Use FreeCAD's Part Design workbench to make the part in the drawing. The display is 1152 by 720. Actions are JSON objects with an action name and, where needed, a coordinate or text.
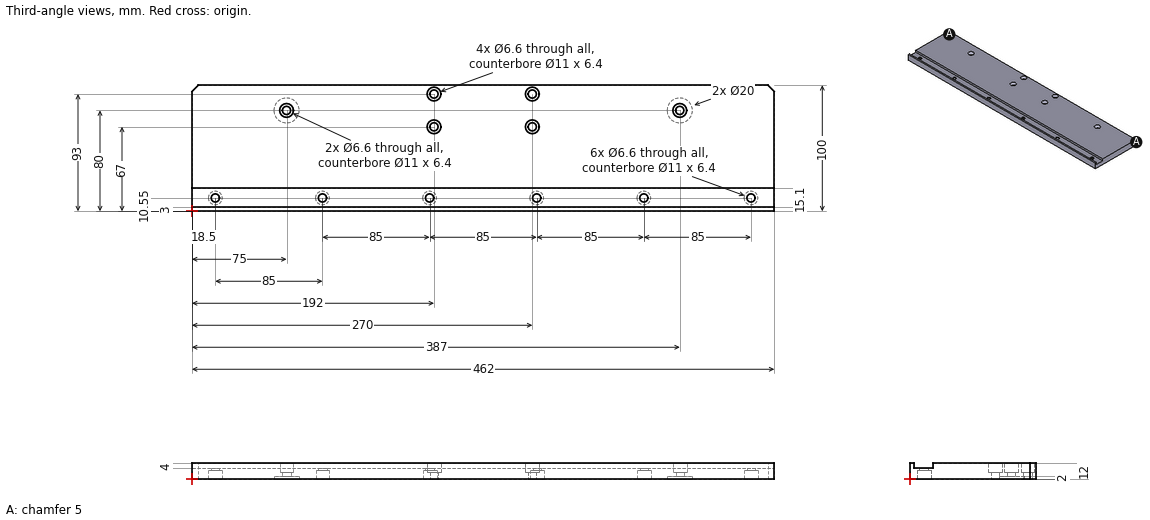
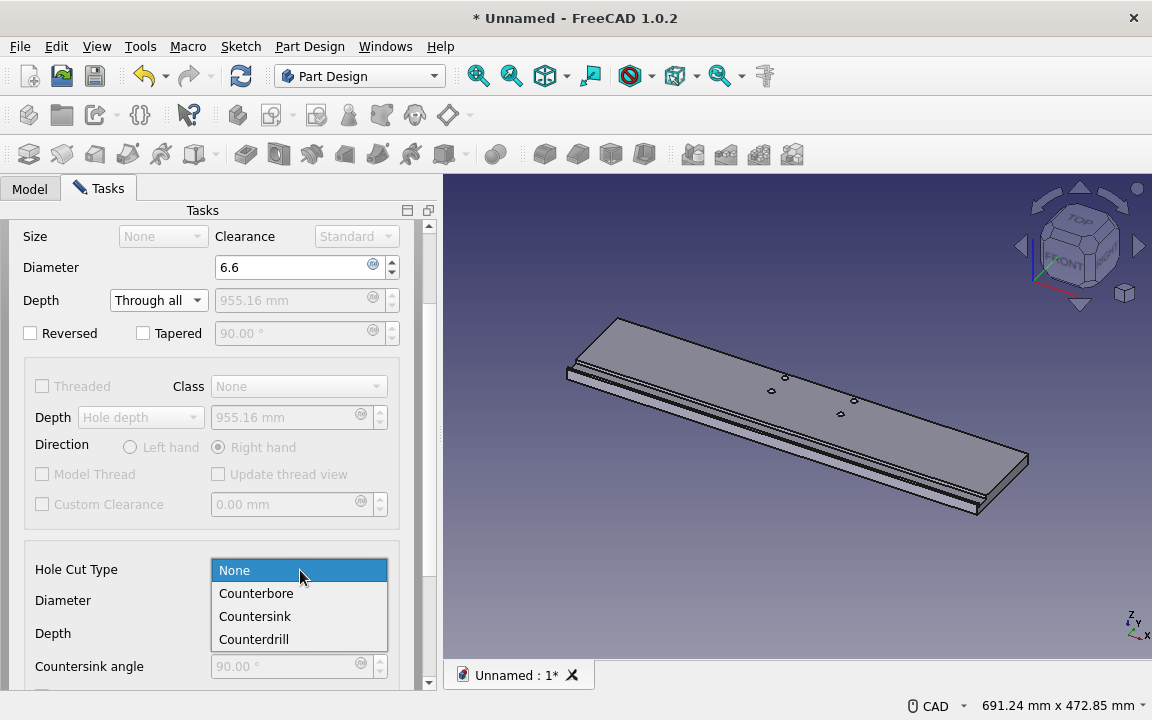
{"action": "left_click", "coordinate": [298, 594]}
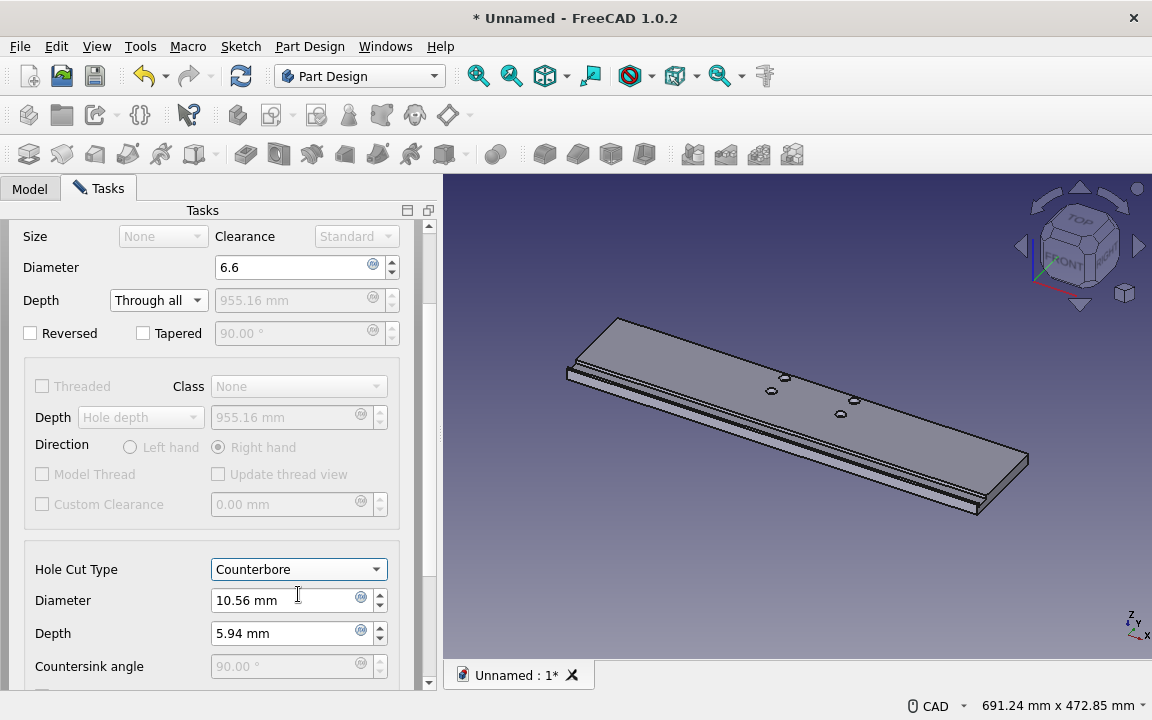
{"action": "triple_click", "coordinate": [292, 600]}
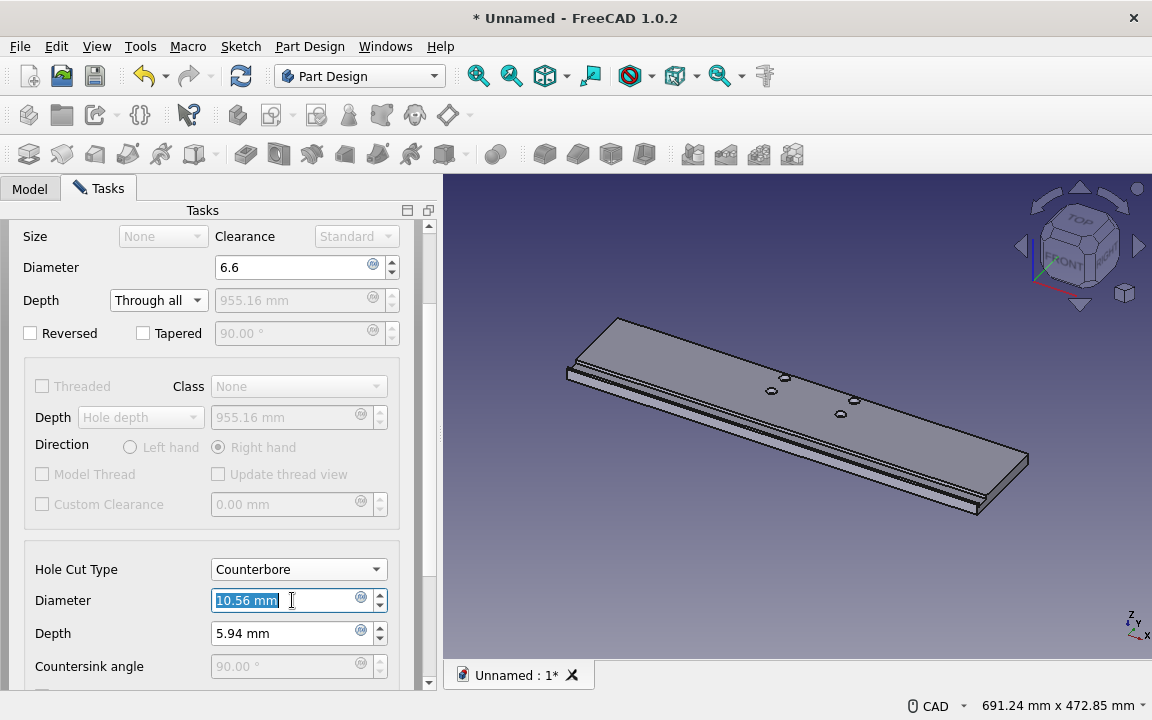
{"action": "type", "text": "11"}
{"action": "key", "text": "Tab"}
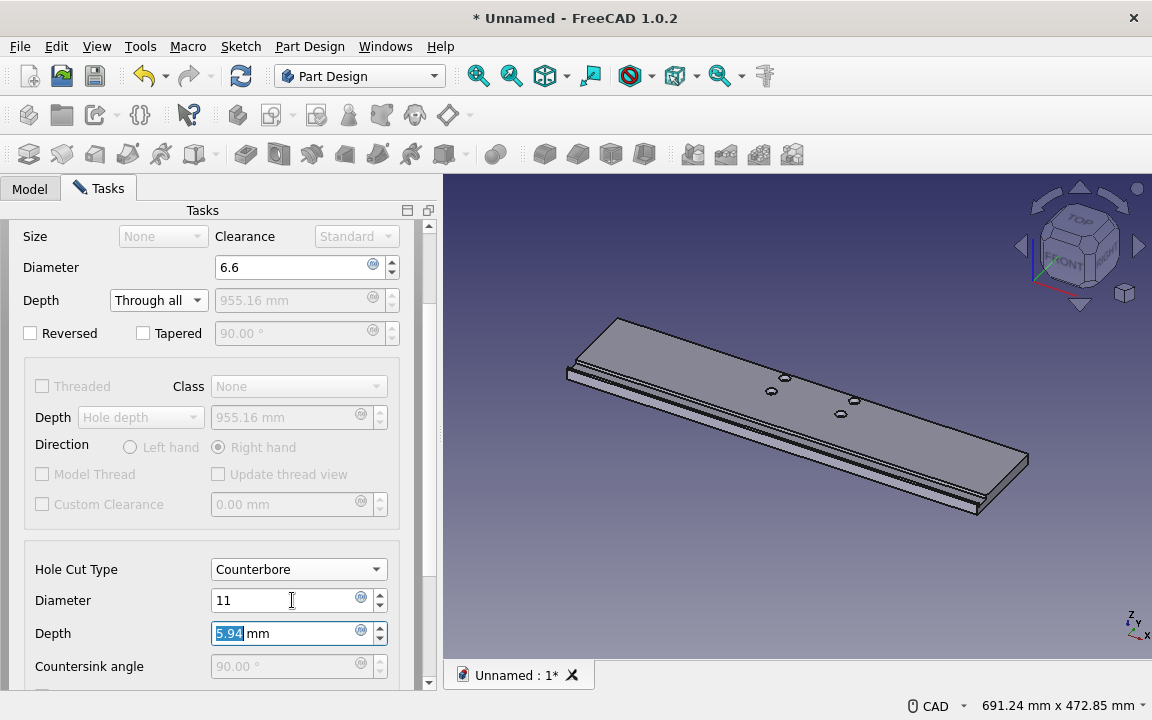
{"action": "type", "text": "6.4"}
{"action": "key", "text": "Tab"}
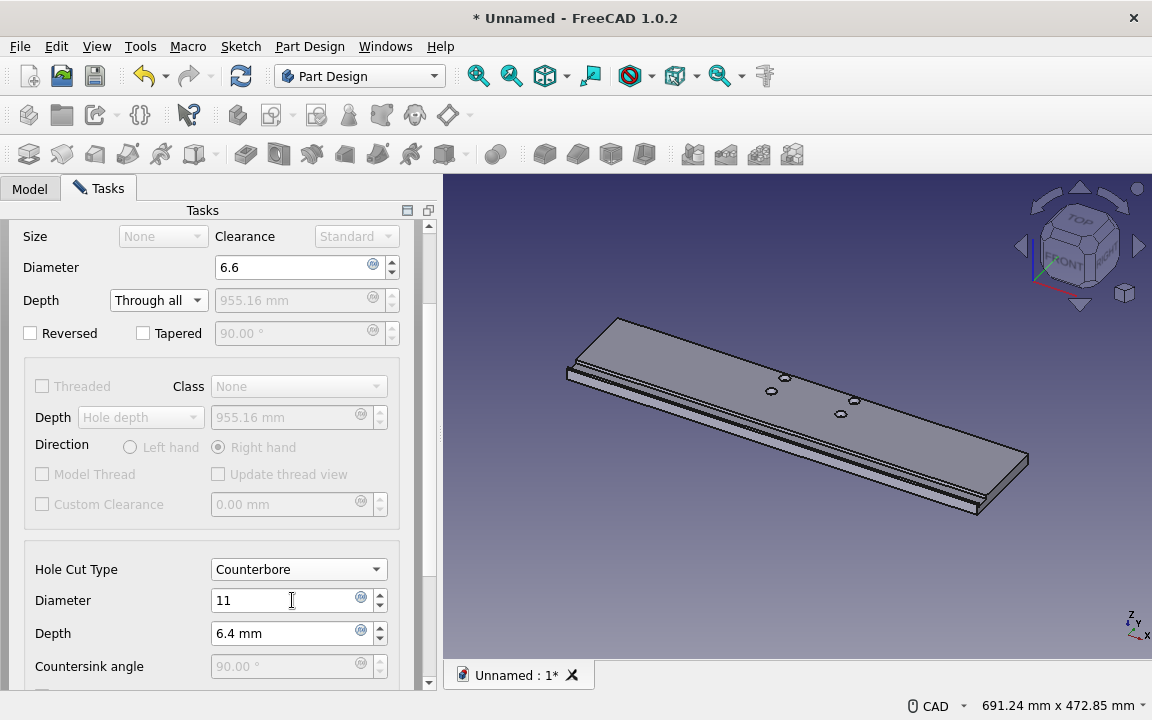
{"action": "scroll", "coordinate": [429, 455], "scroll_direction": "up", "scroll_amount": 3}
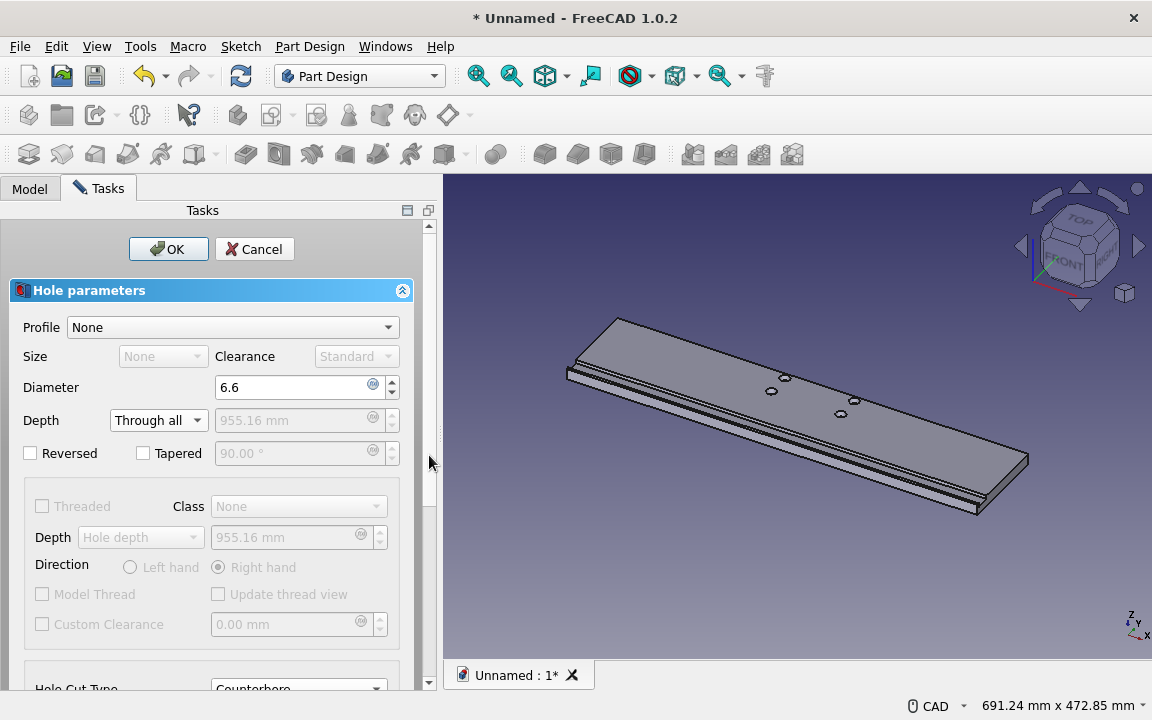
{"action": "left_click", "coordinate": [169, 249]}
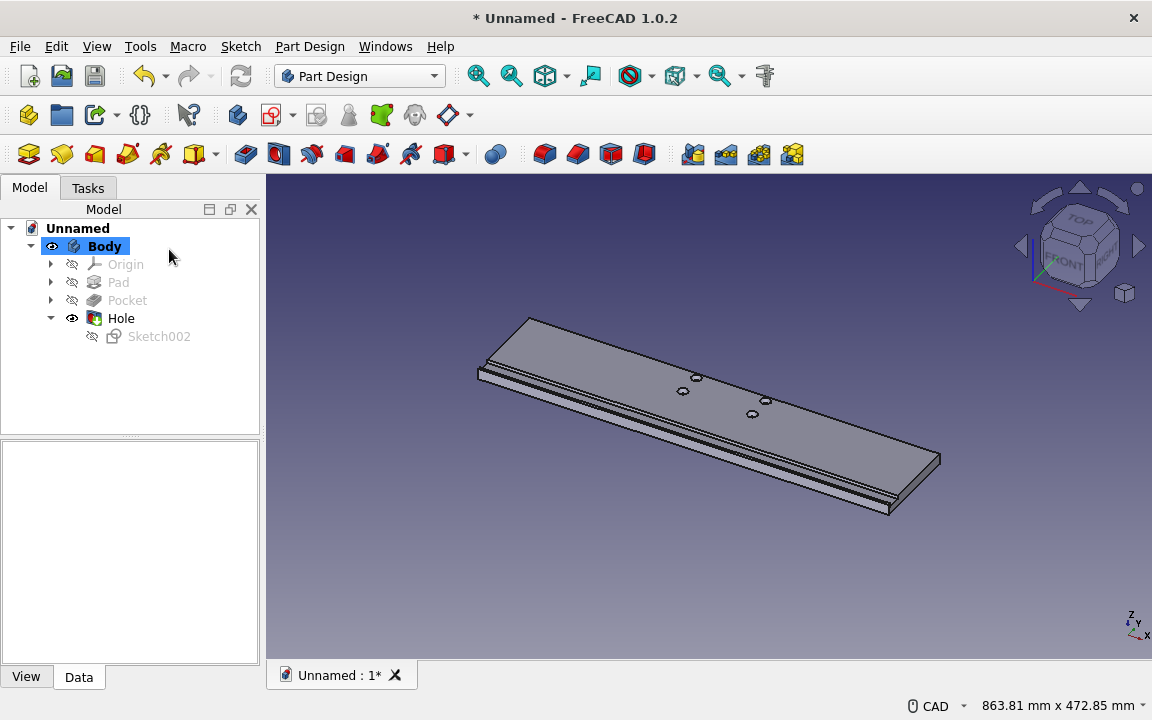
{"action": "left_click", "coordinate": [270, 116]}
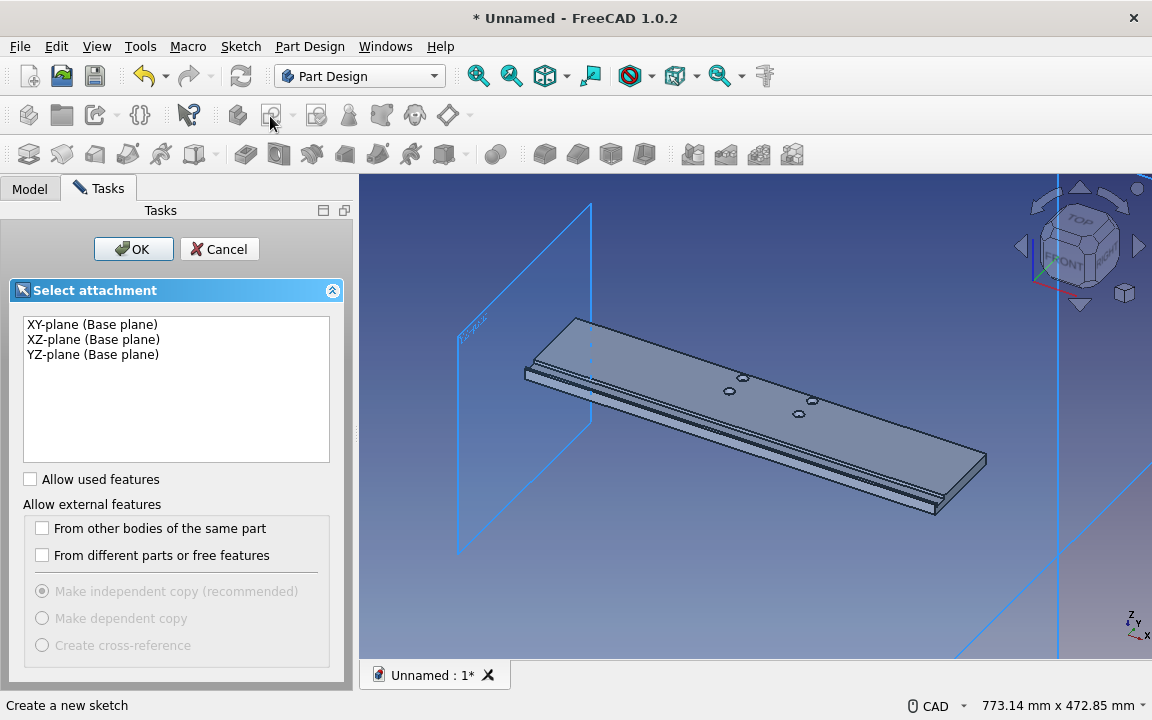
{"action": "left_click", "coordinate": [84, 324]}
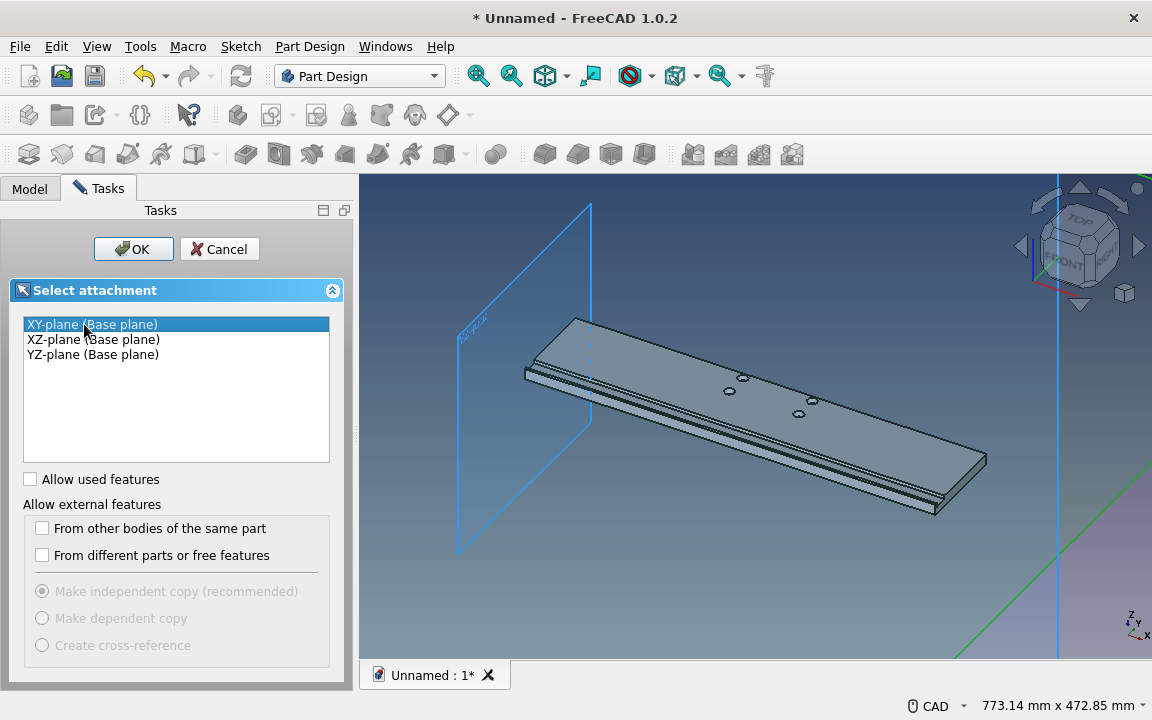
{"action": "left_click", "coordinate": [134, 249]}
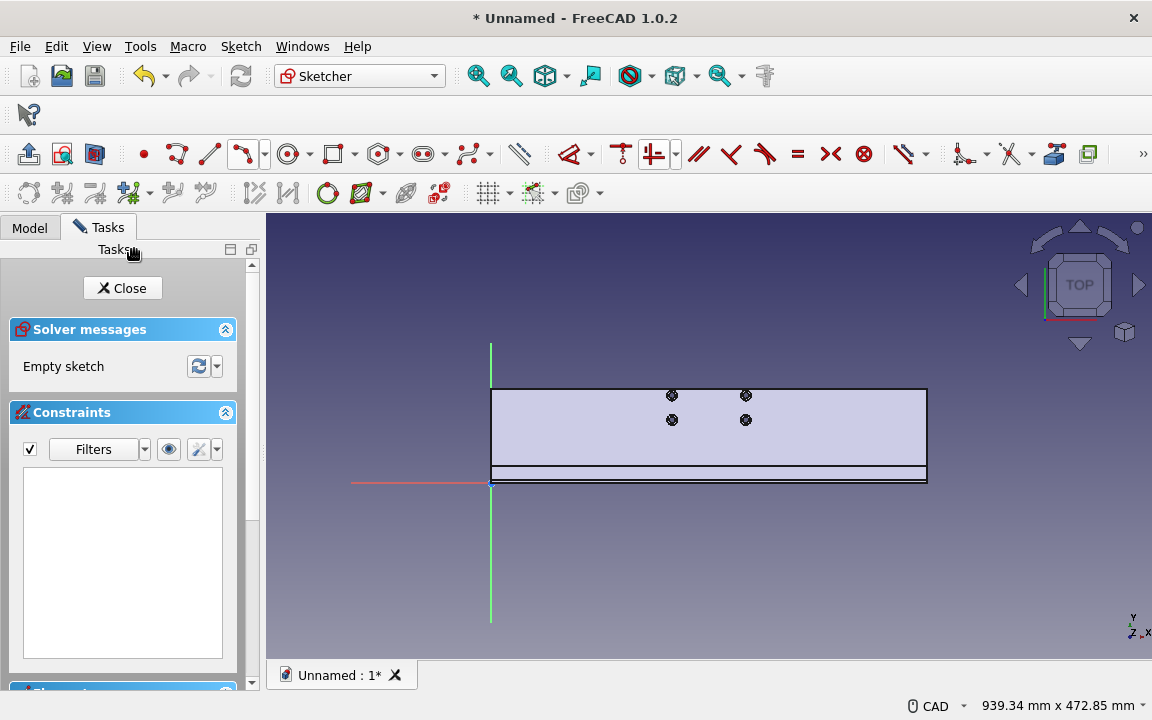
{"action": "left_click", "coordinate": [95, 154]}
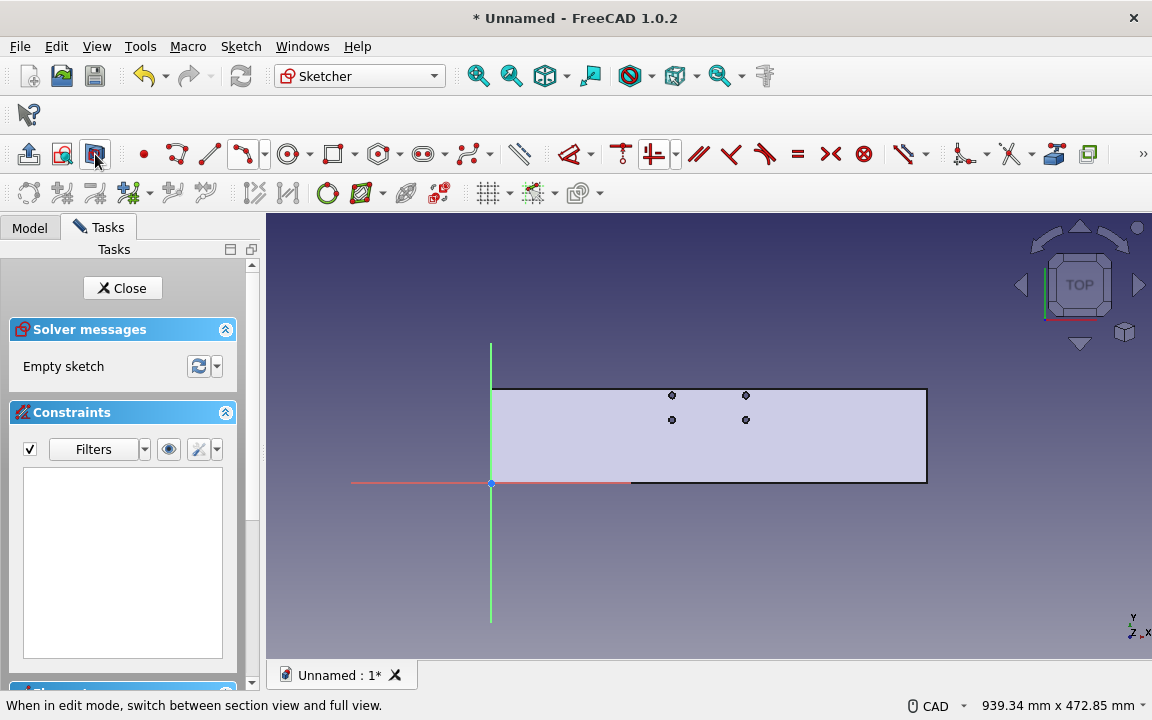
{"action": "left_click", "coordinate": [288, 154]}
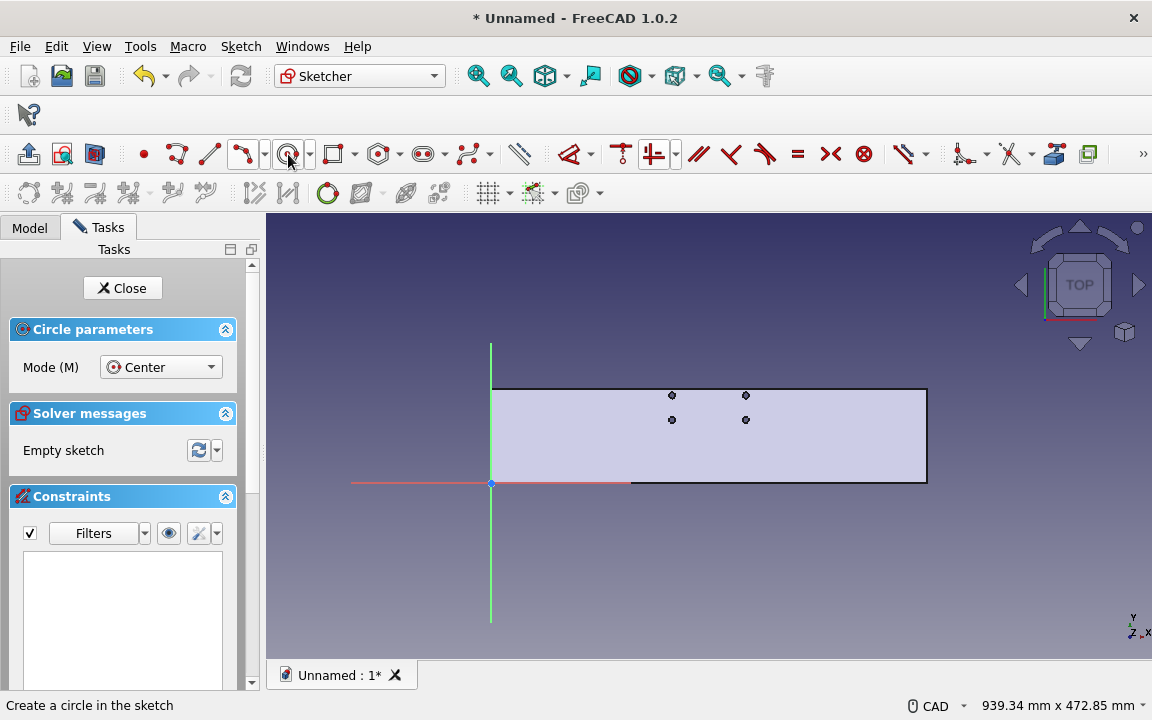
{"action": "scroll", "coordinate": [856, 408], "scroll_direction": "up", "scroll_amount": 5}